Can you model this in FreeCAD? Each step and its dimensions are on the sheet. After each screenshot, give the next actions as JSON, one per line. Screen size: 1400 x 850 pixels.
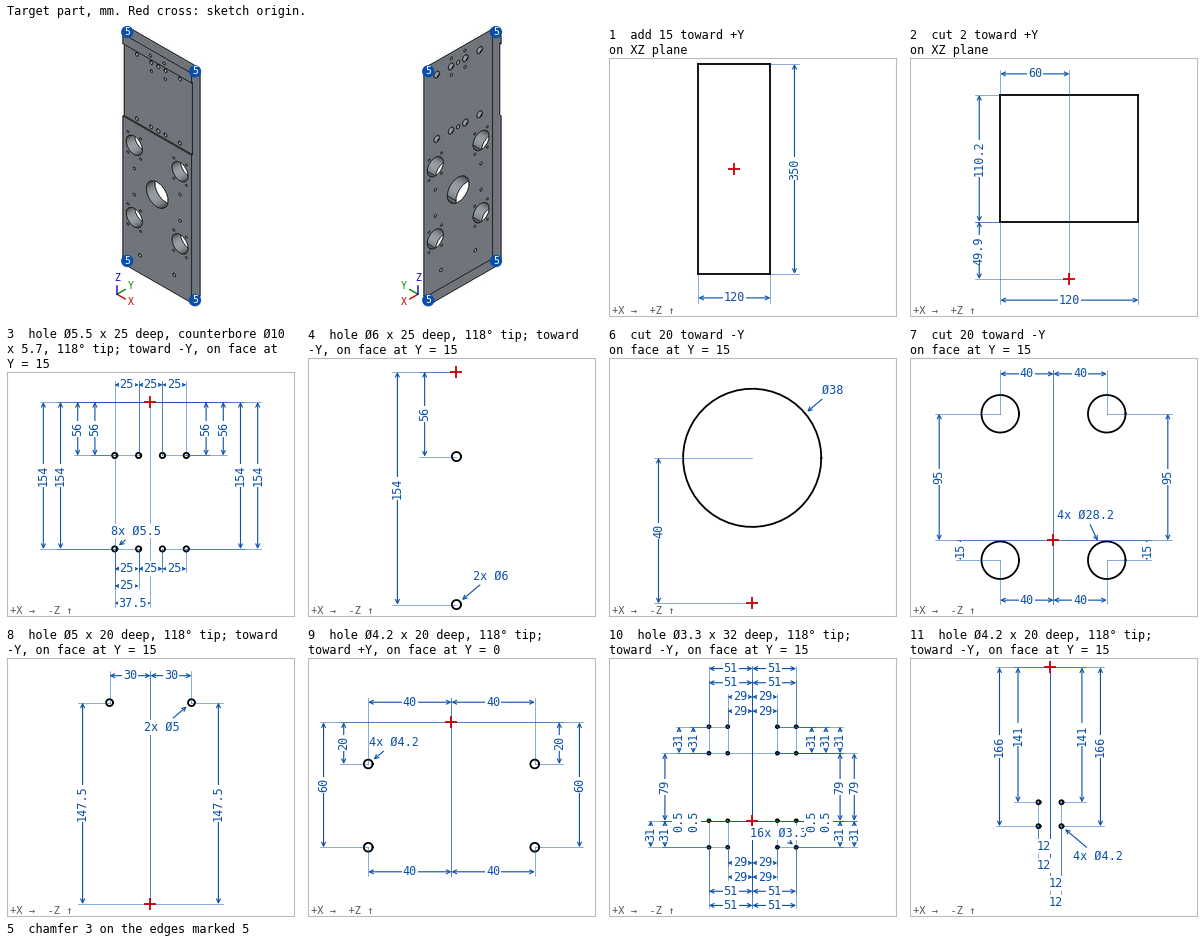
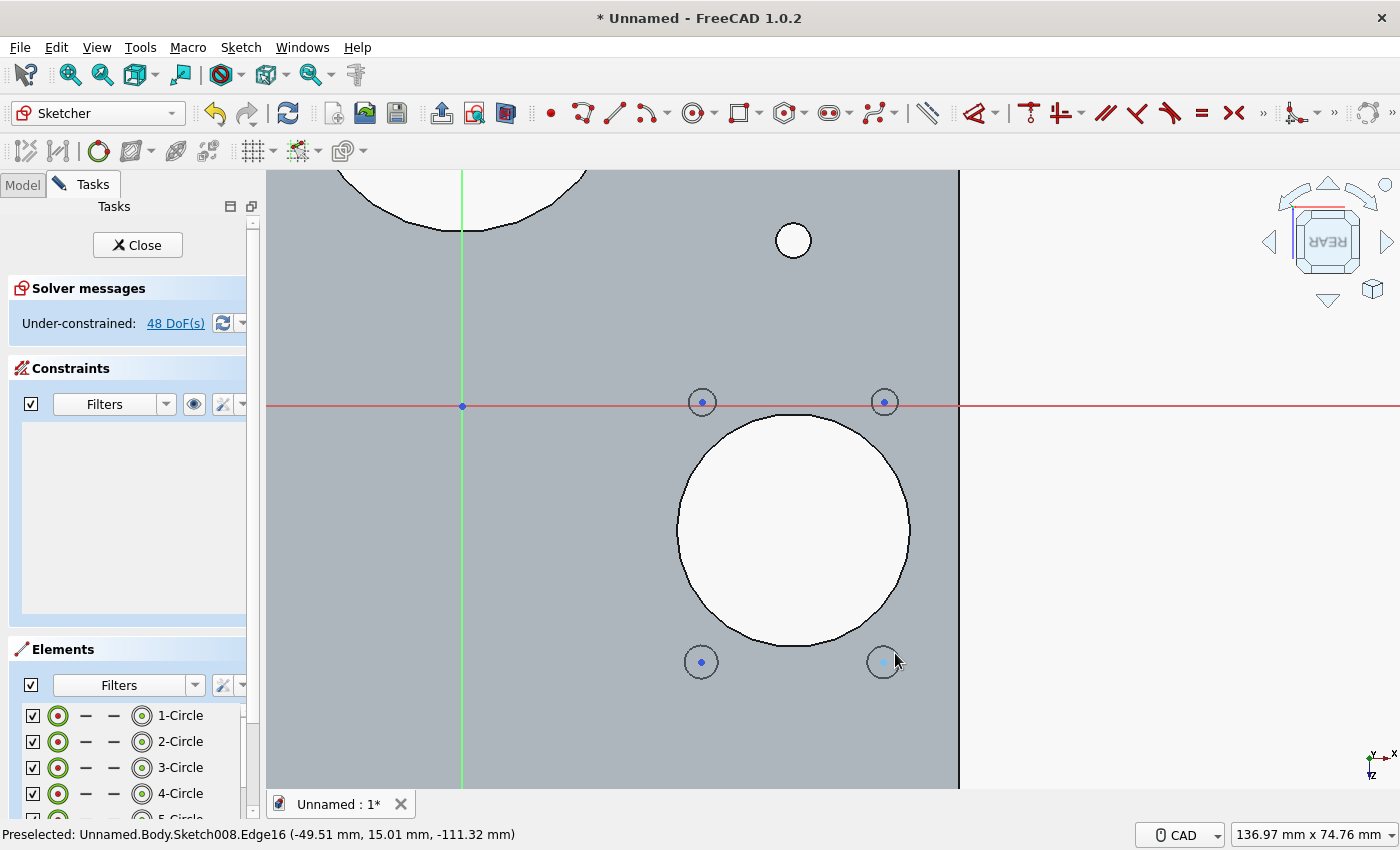
{"action": "left_click", "coordinate": [895, 651]}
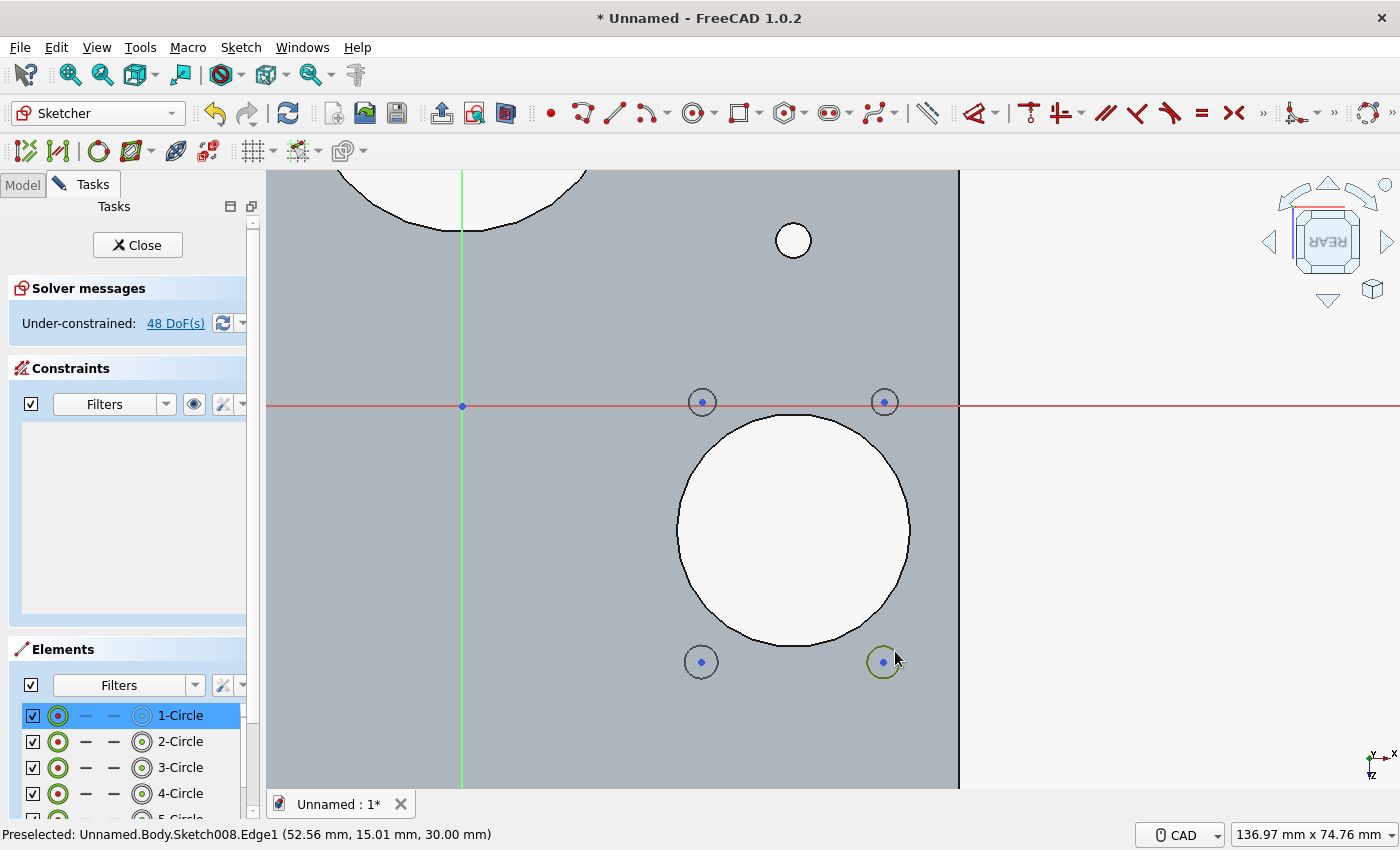
{"action": "left_click", "coordinate": [713, 650]}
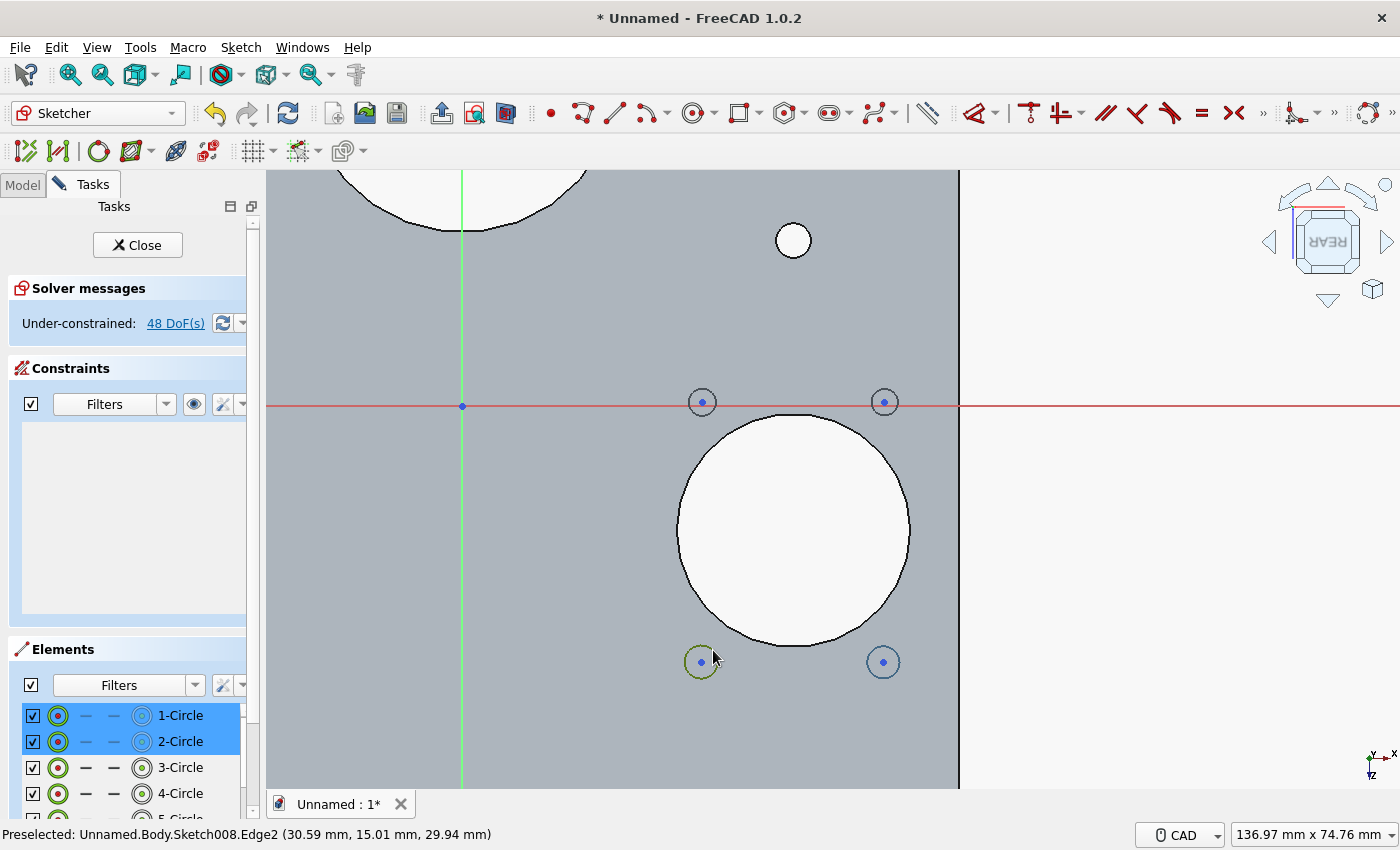
{"action": "left_click", "coordinate": [894, 393]}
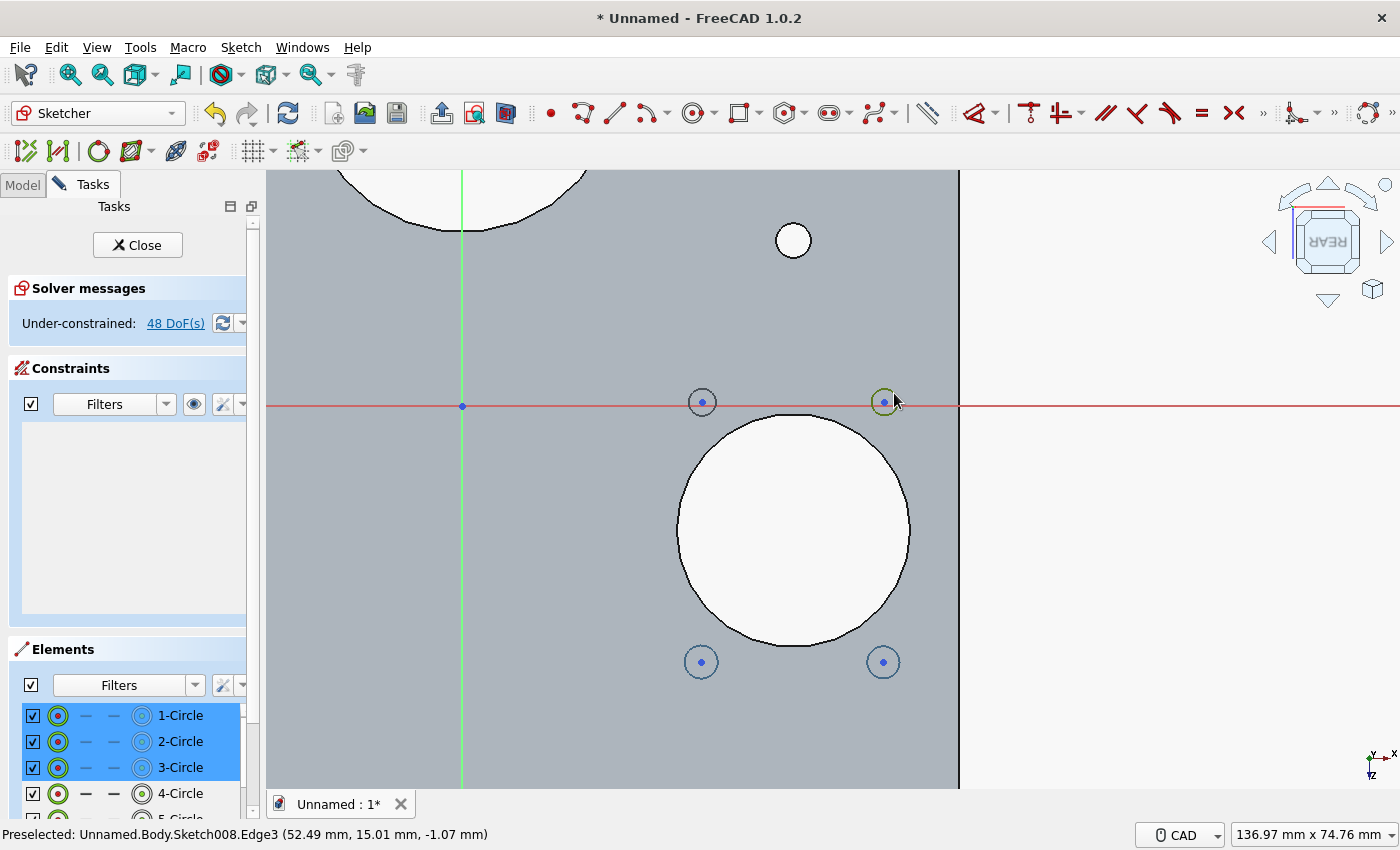
{"action": "left_click", "coordinate": [712, 393]}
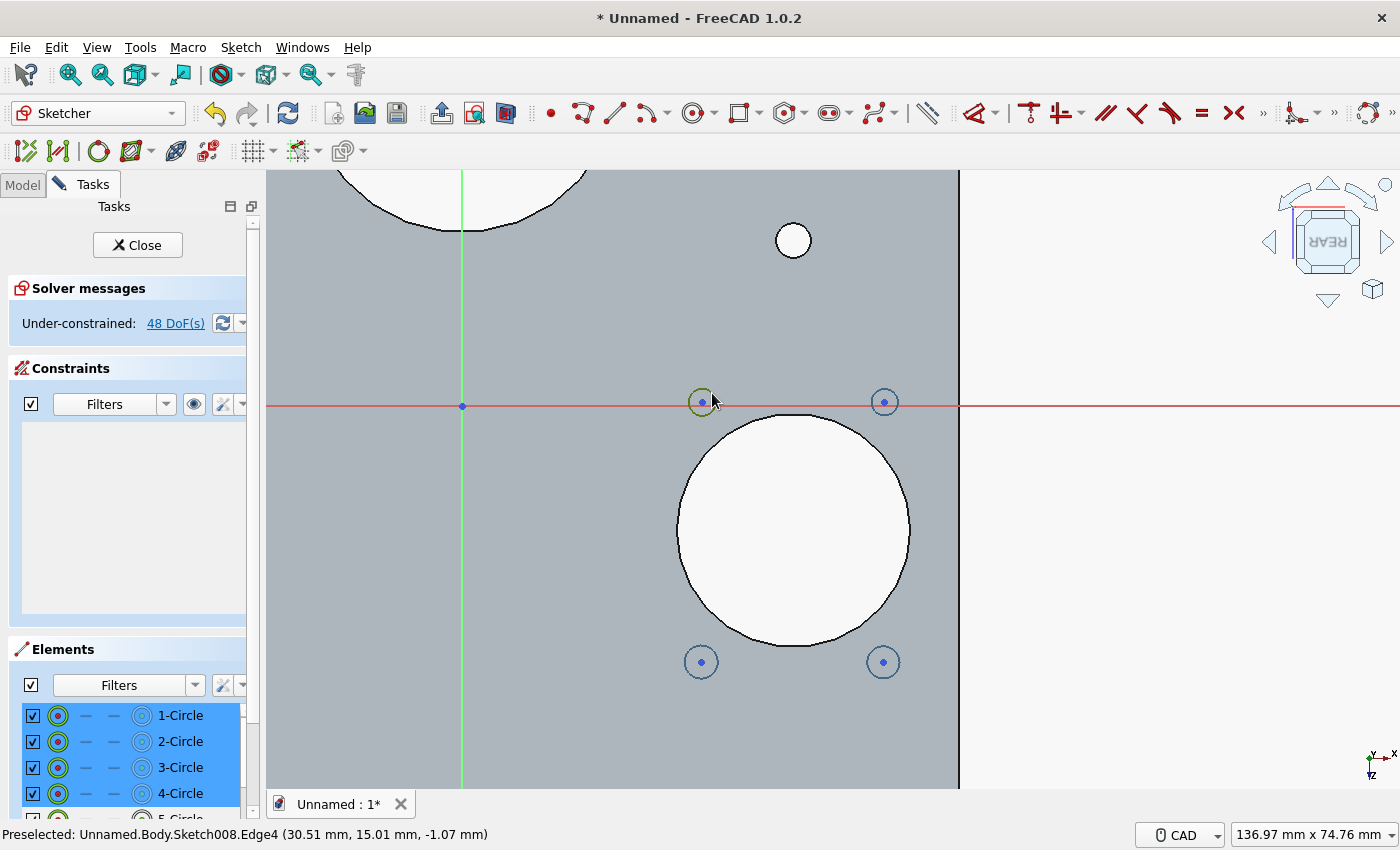
{"action": "scroll", "coordinate": [895, 654], "scroll_direction": "down", "scroll_amount": 6}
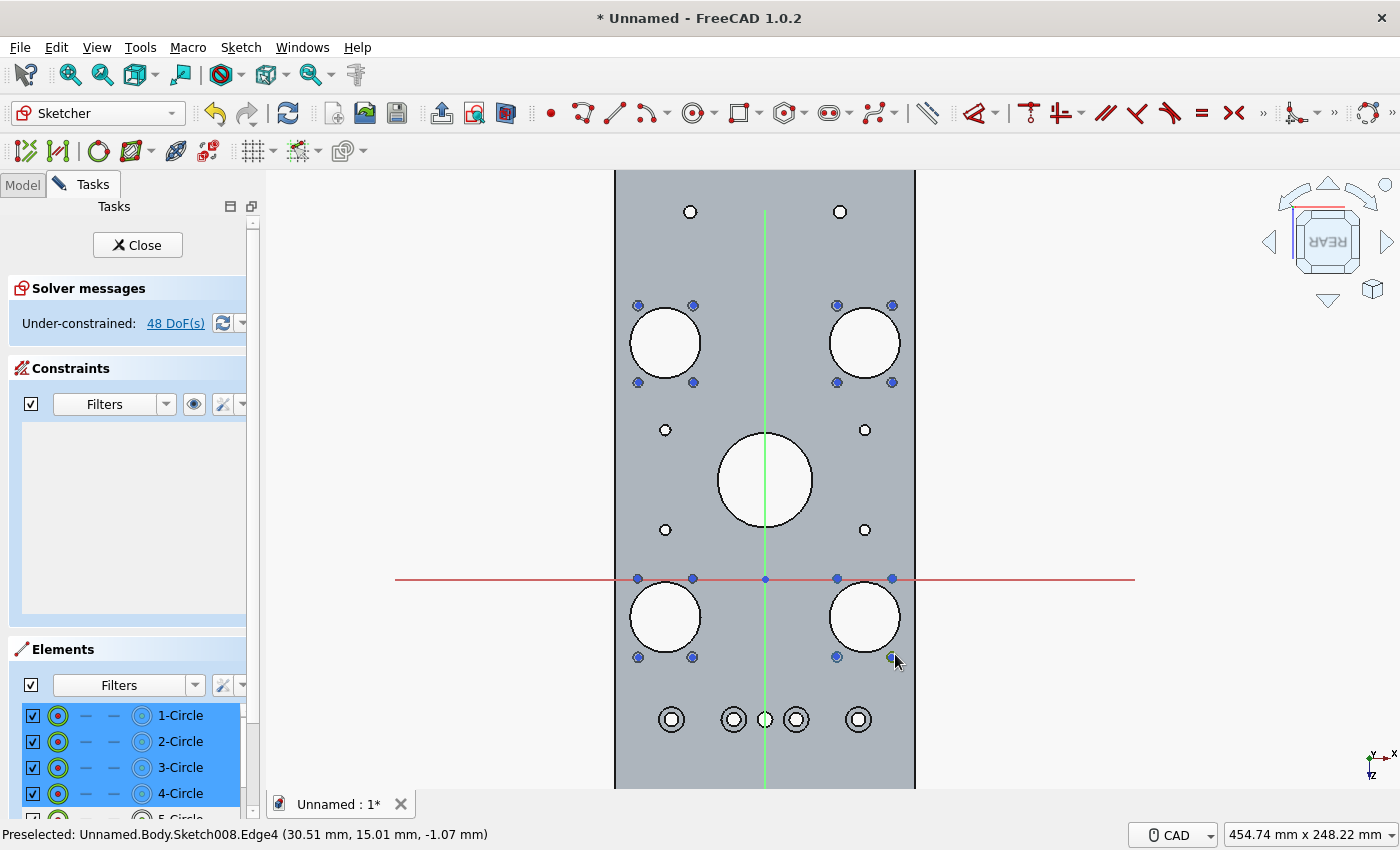
{"action": "scroll", "coordinate": [642, 654], "scroll_direction": "up", "scroll_amount": 6}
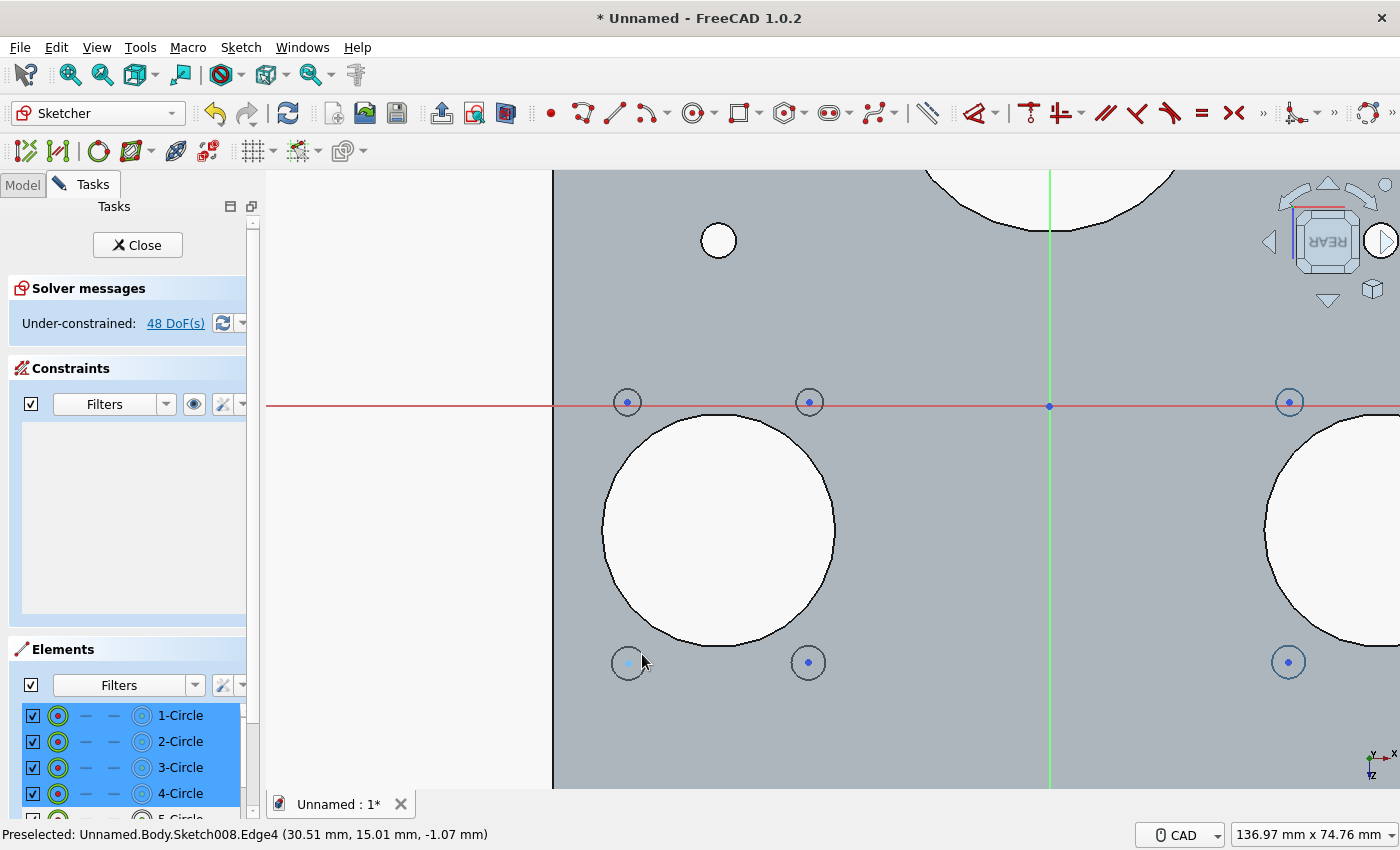
{"action": "left_click", "coordinate": [640, 652]}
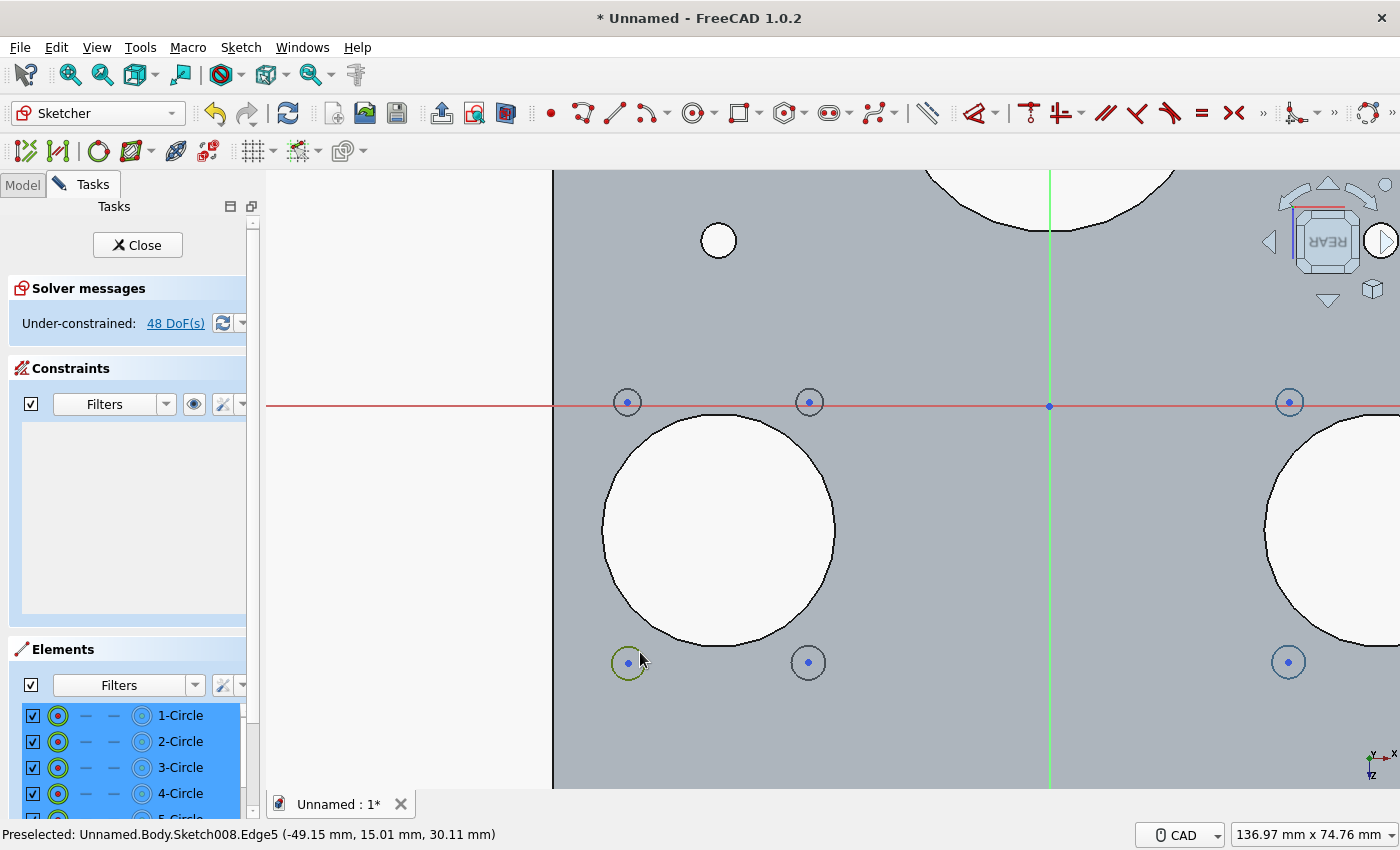
{"action": "left_click", "coordinate": [820, 651]}